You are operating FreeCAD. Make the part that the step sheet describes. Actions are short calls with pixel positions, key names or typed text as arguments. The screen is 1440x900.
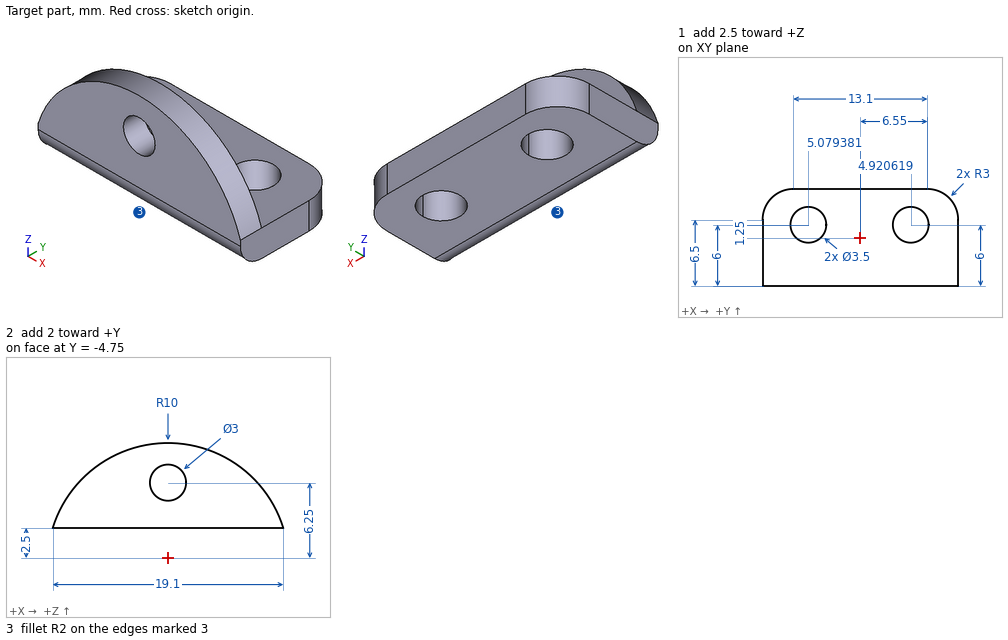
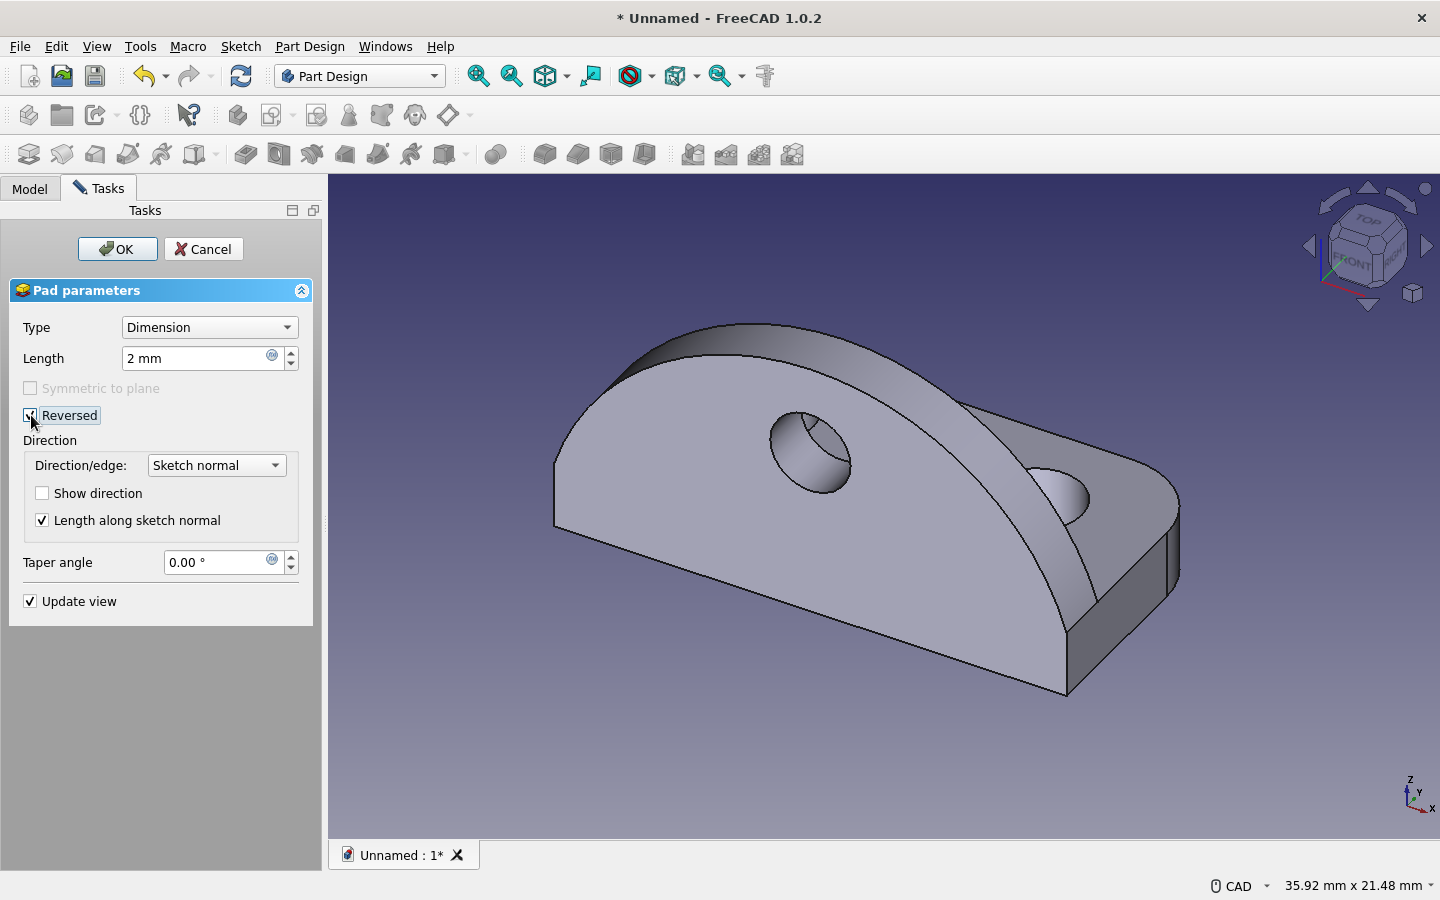
click(118, 249)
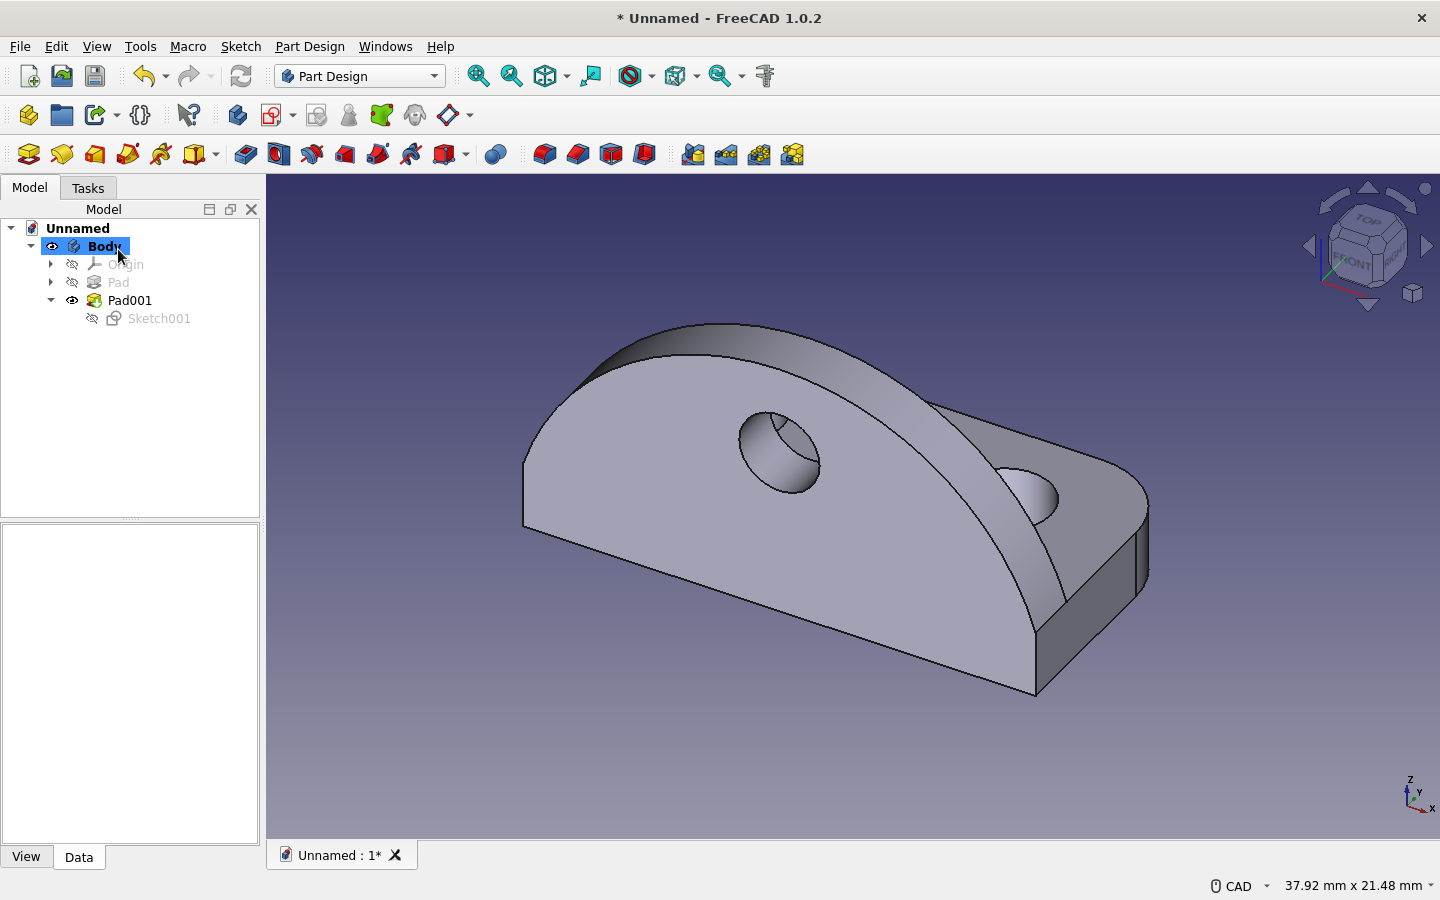
click(479, 76)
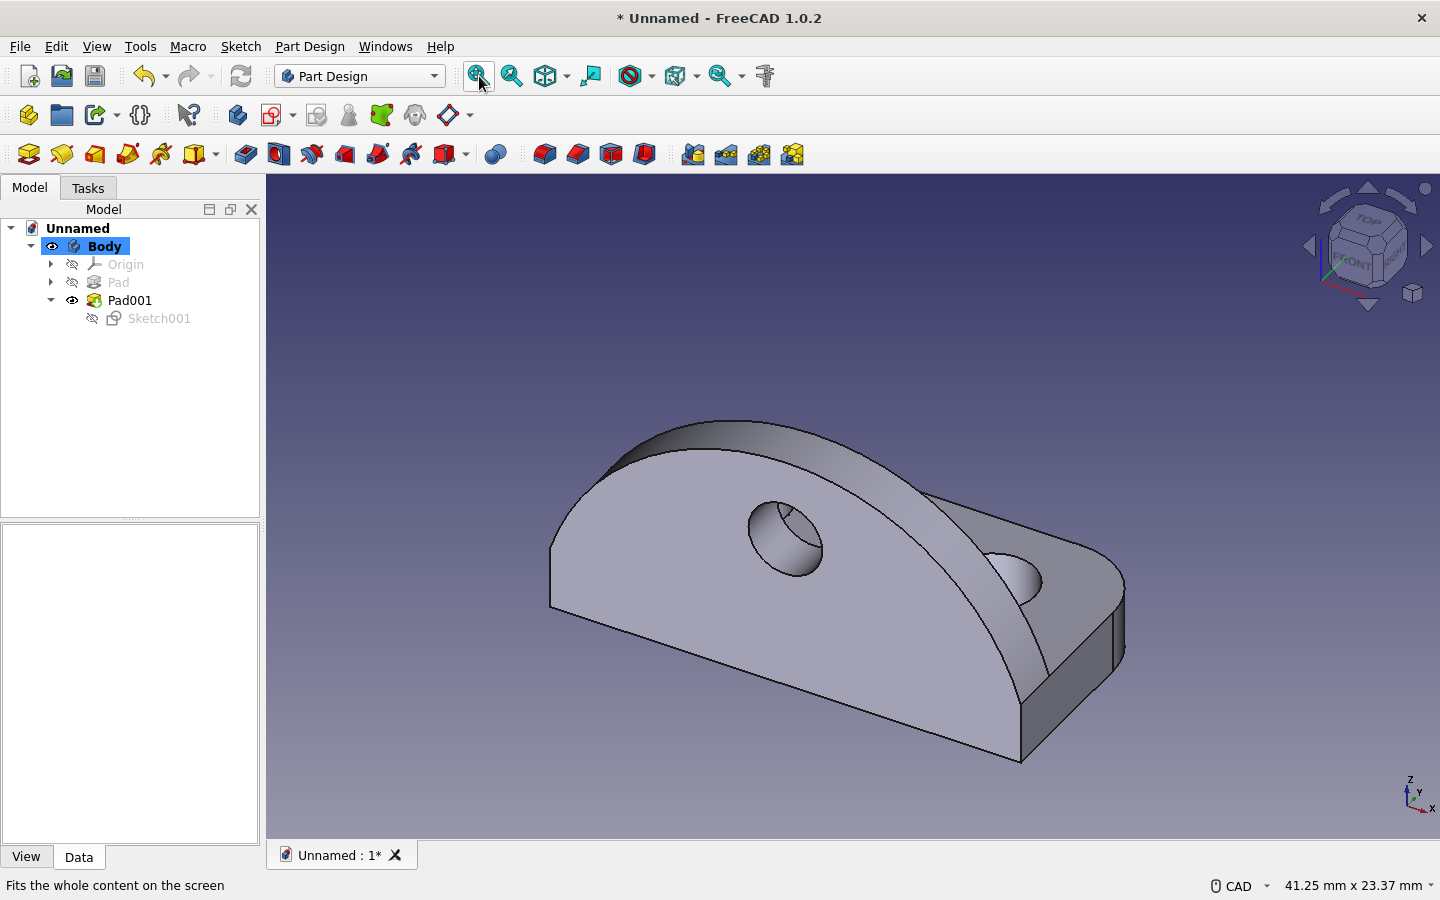
key(0)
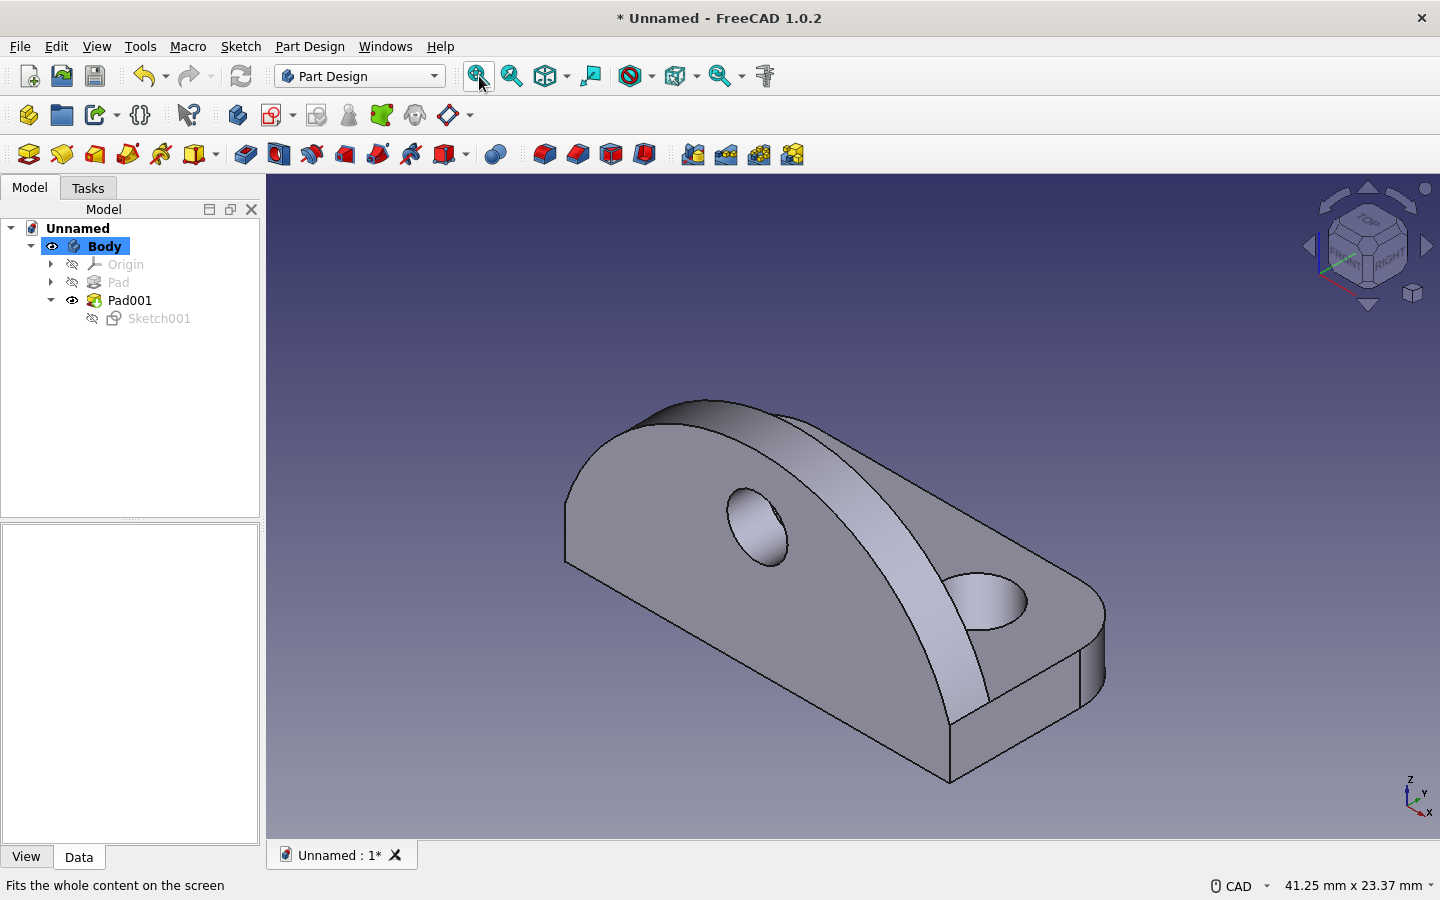
key(2)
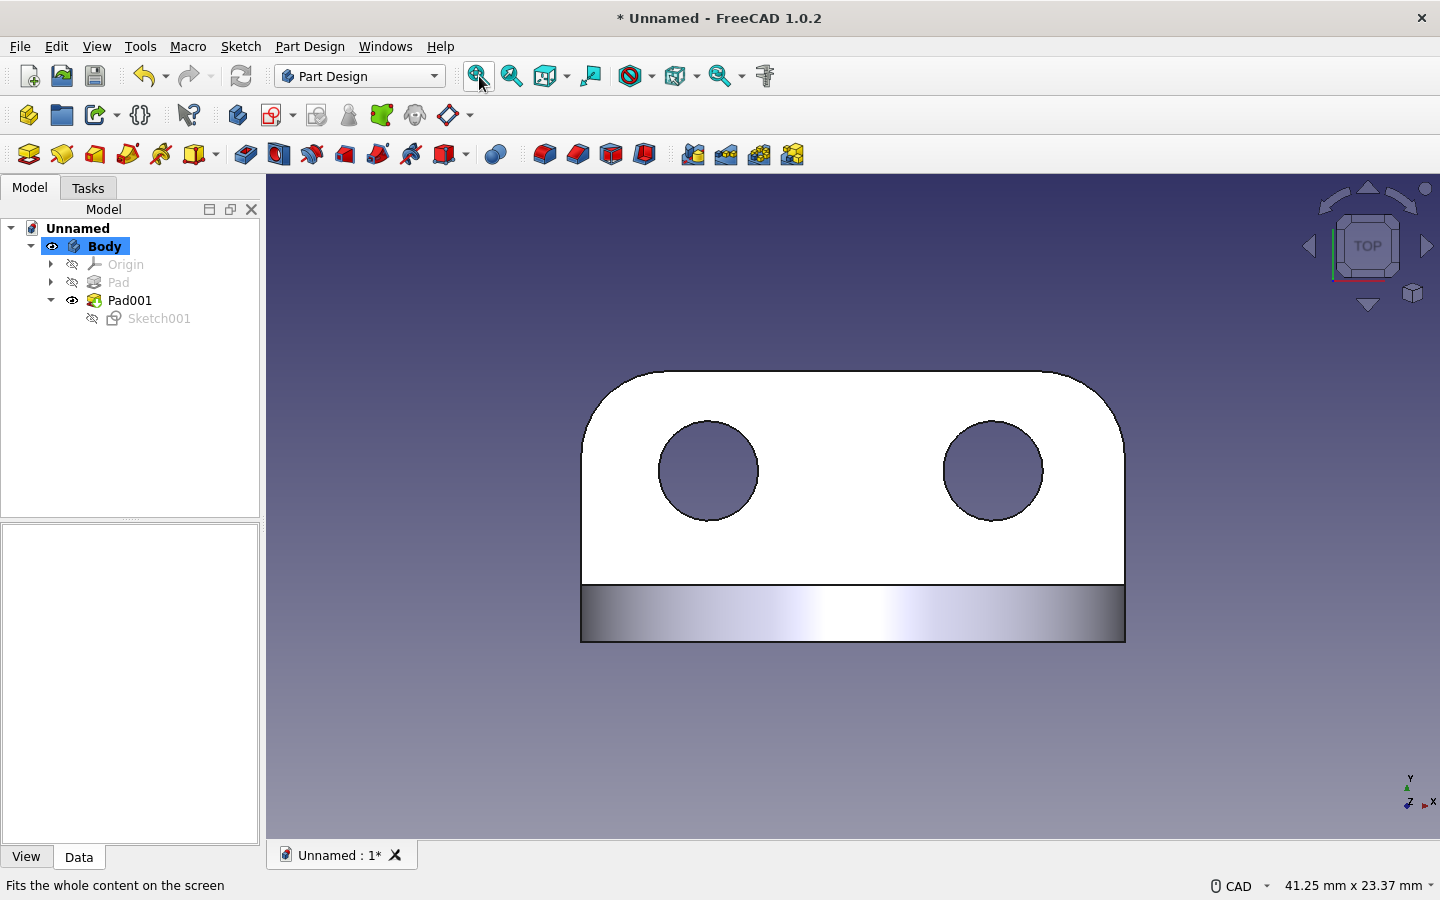
key(1)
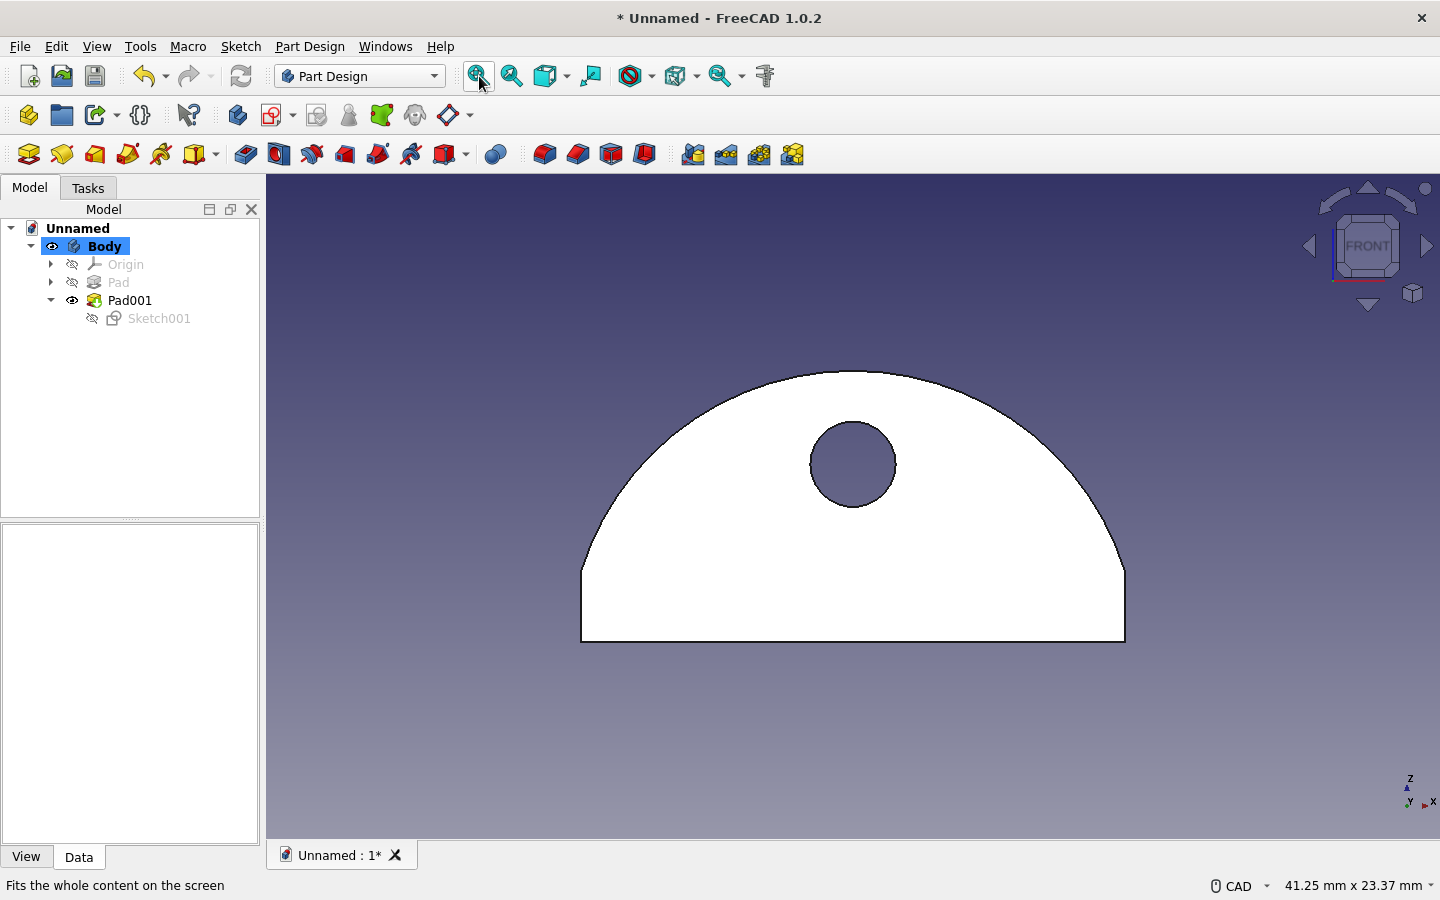
click(853, 641)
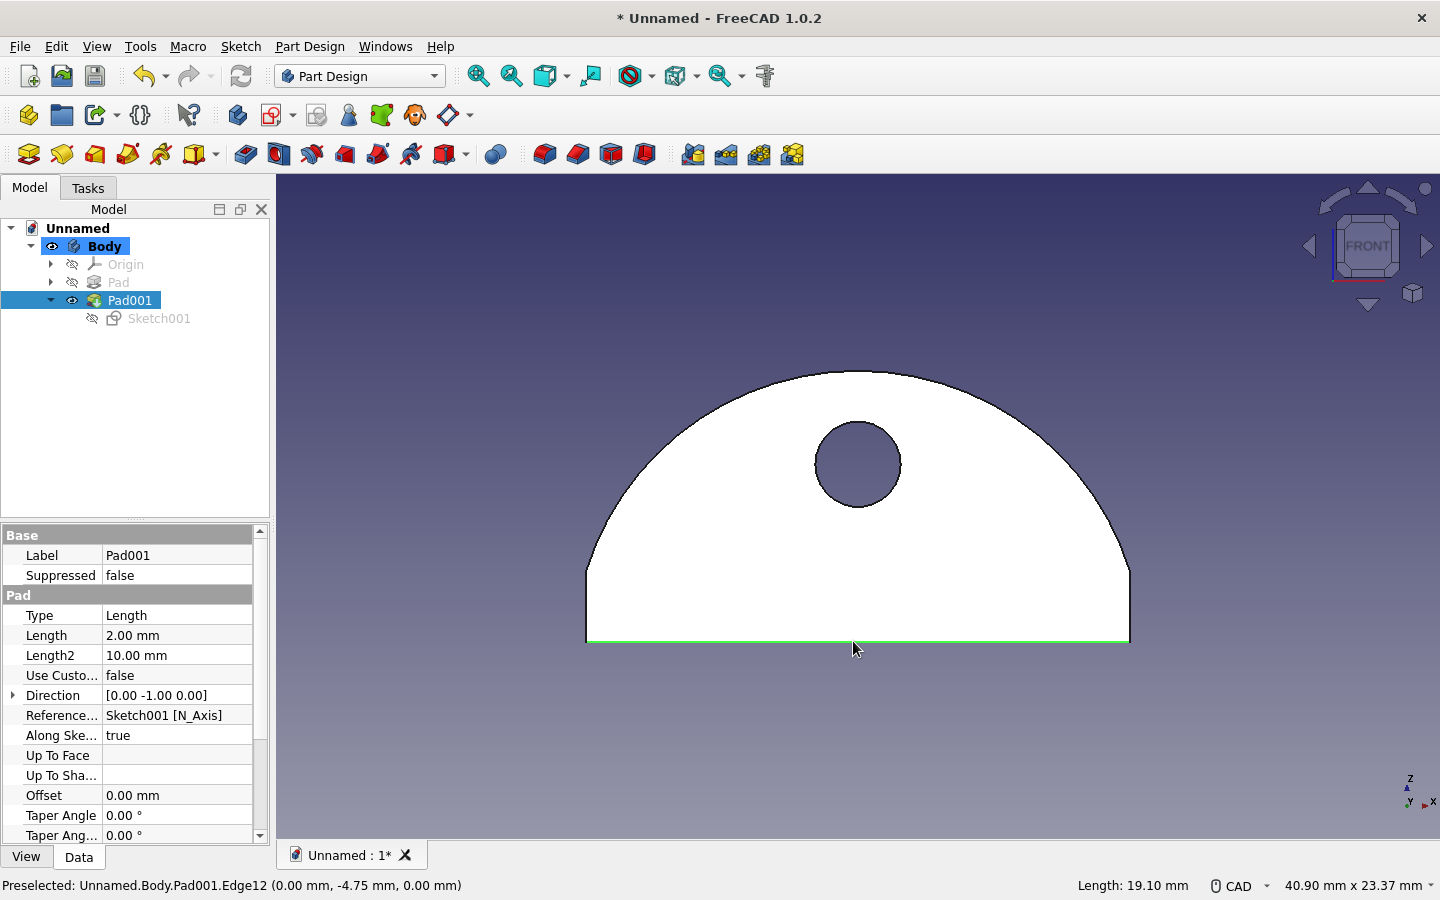
click(545, 154)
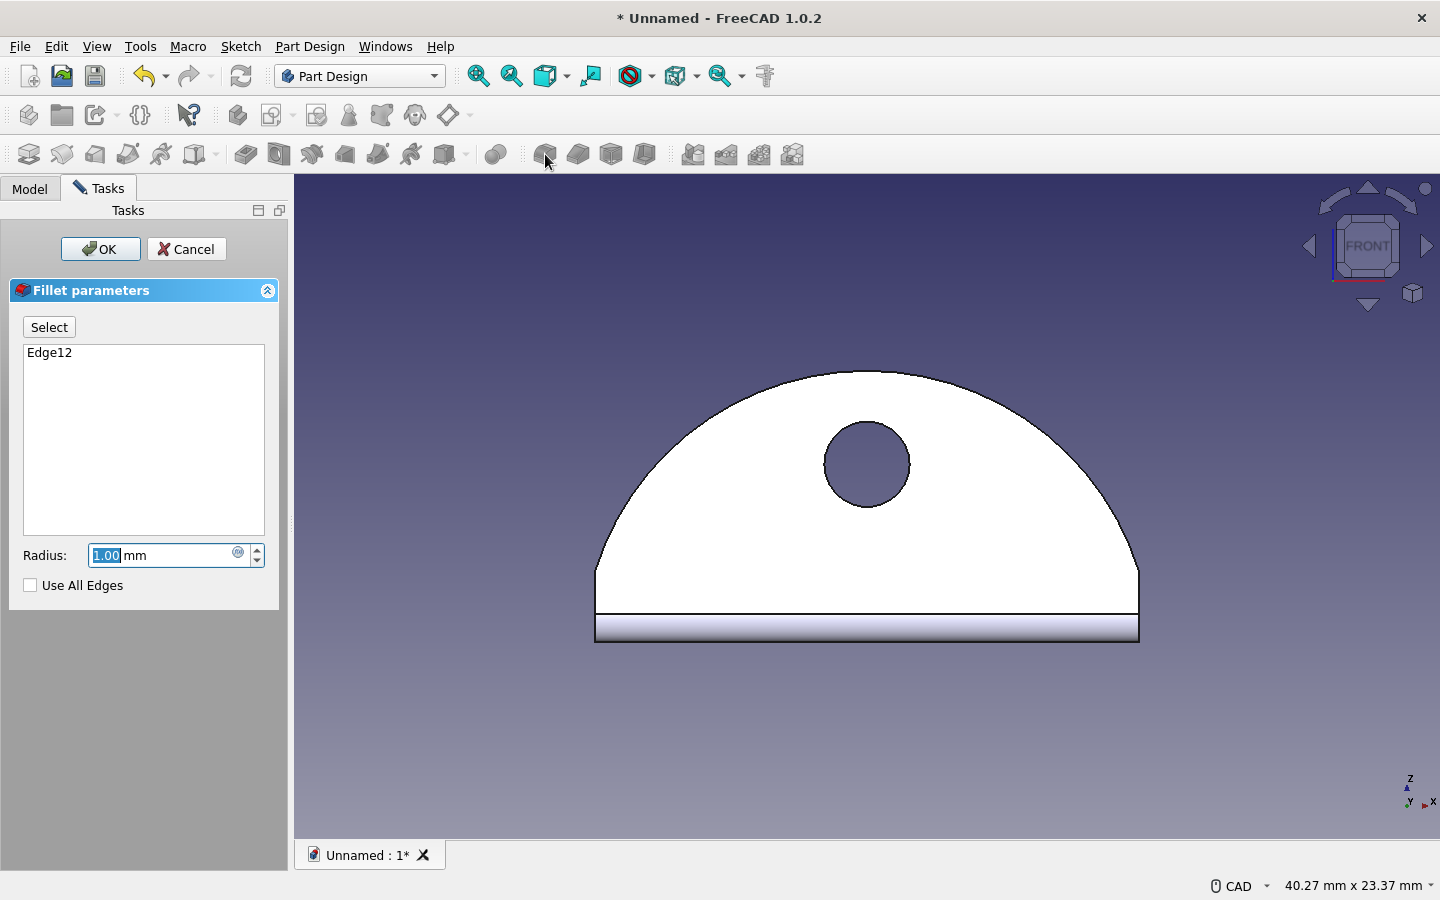
text(2)
key(Tab)